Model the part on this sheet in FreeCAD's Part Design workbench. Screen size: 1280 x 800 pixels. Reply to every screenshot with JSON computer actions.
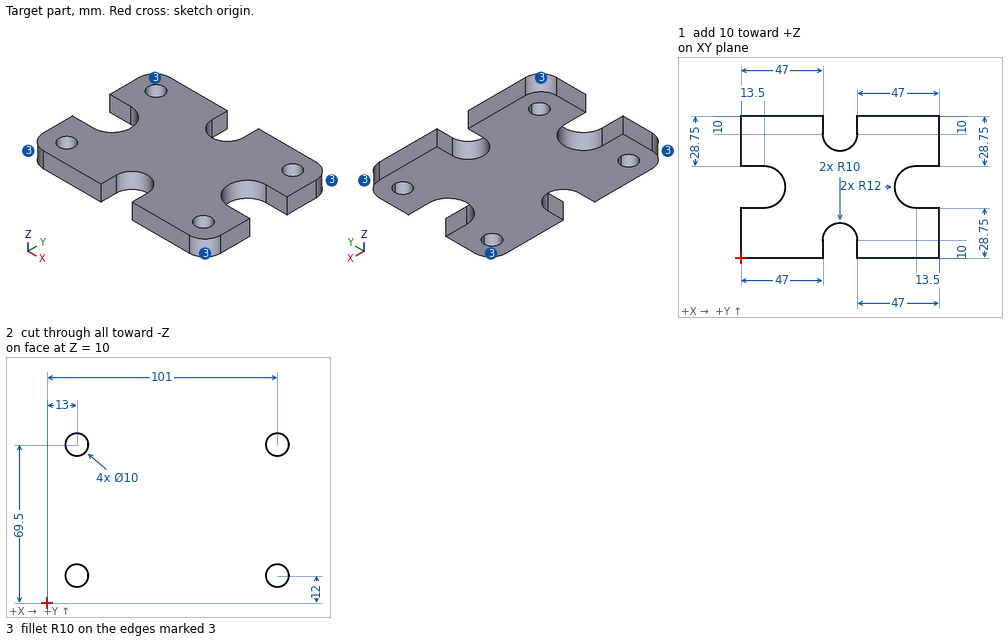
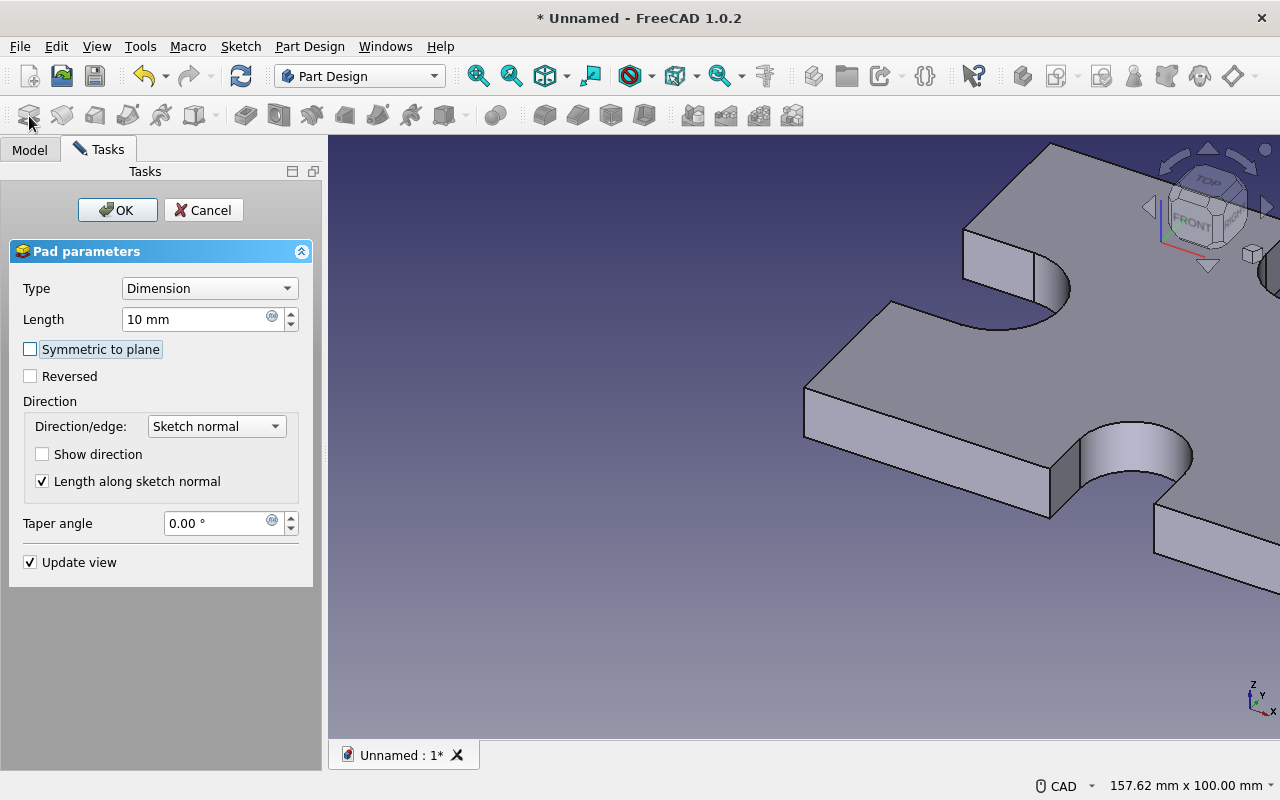
{"action": "left_click", "coordinate": [118, 210]}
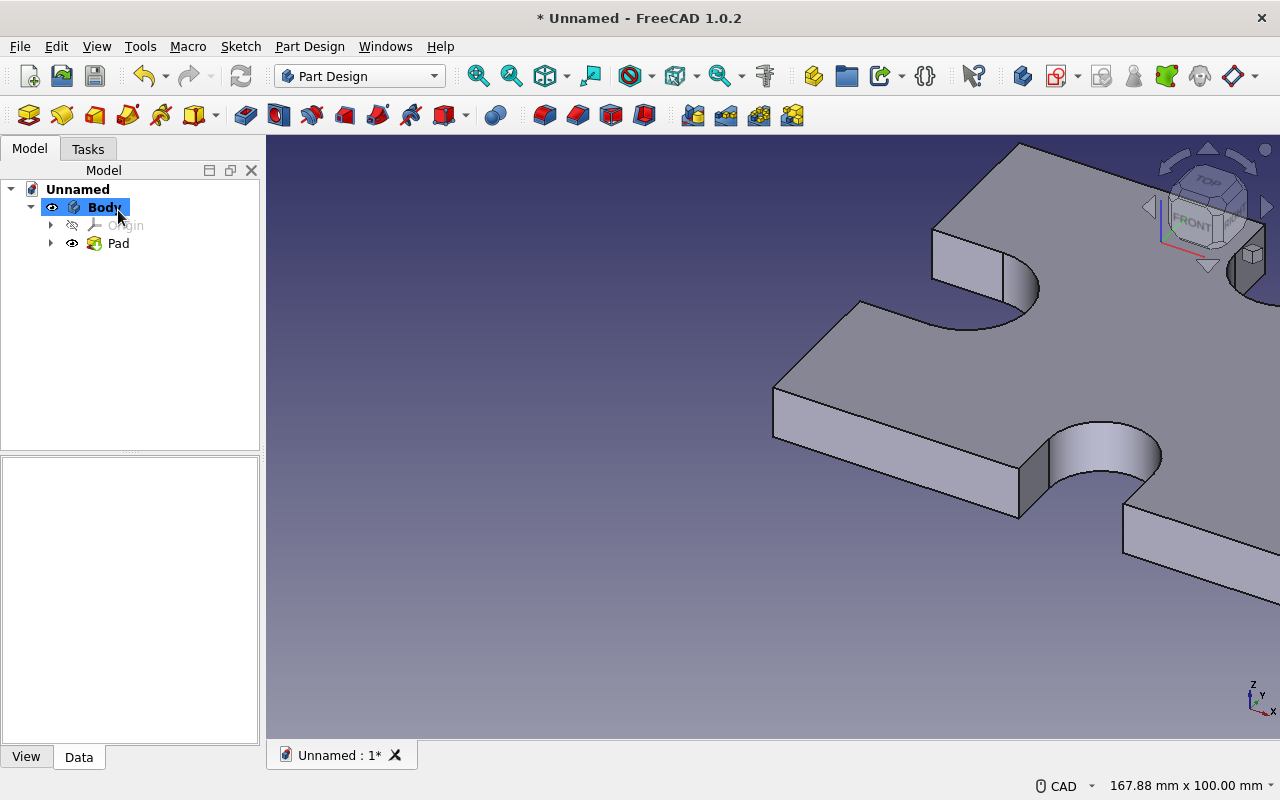
{"action": "left_click", "coordinate": [479, 76]}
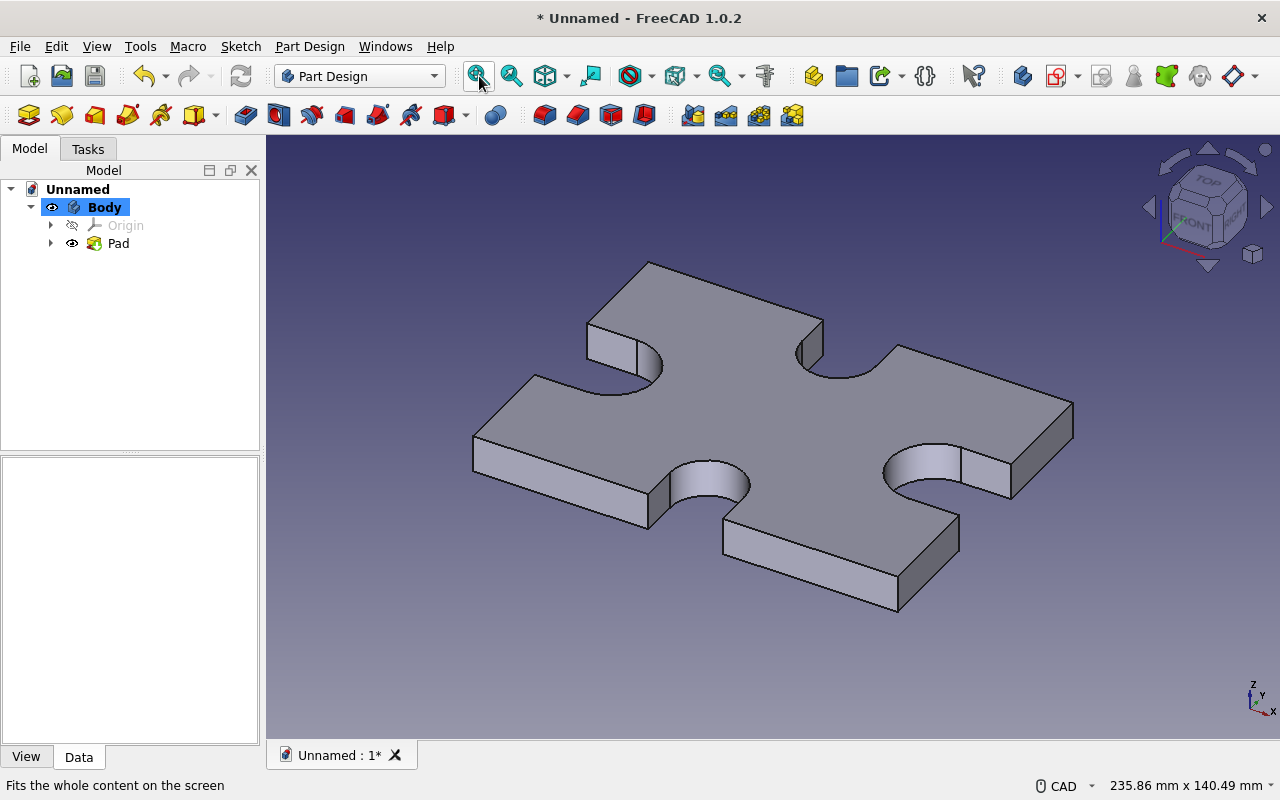
{"action": "left_click", "coordinate": [773, 418]}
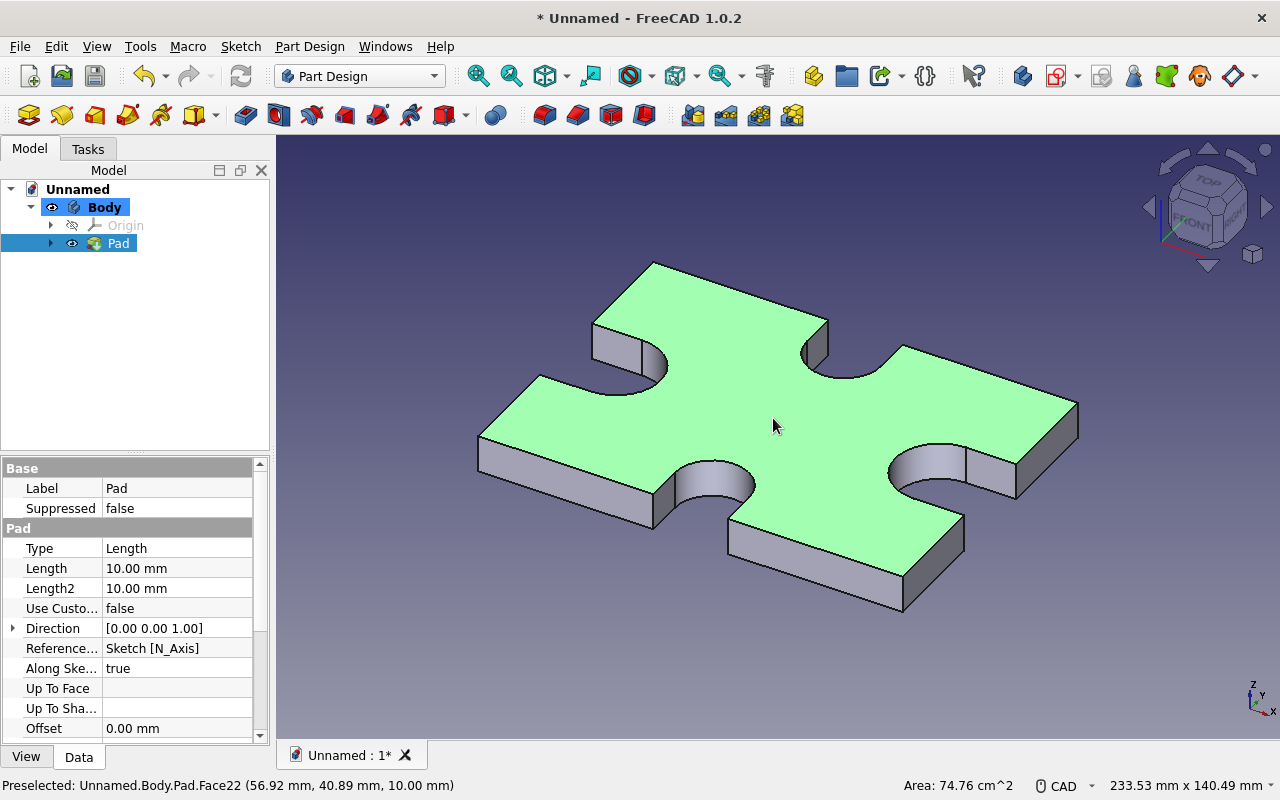
{"action": "left_click", "coordinate": [1056, 76]}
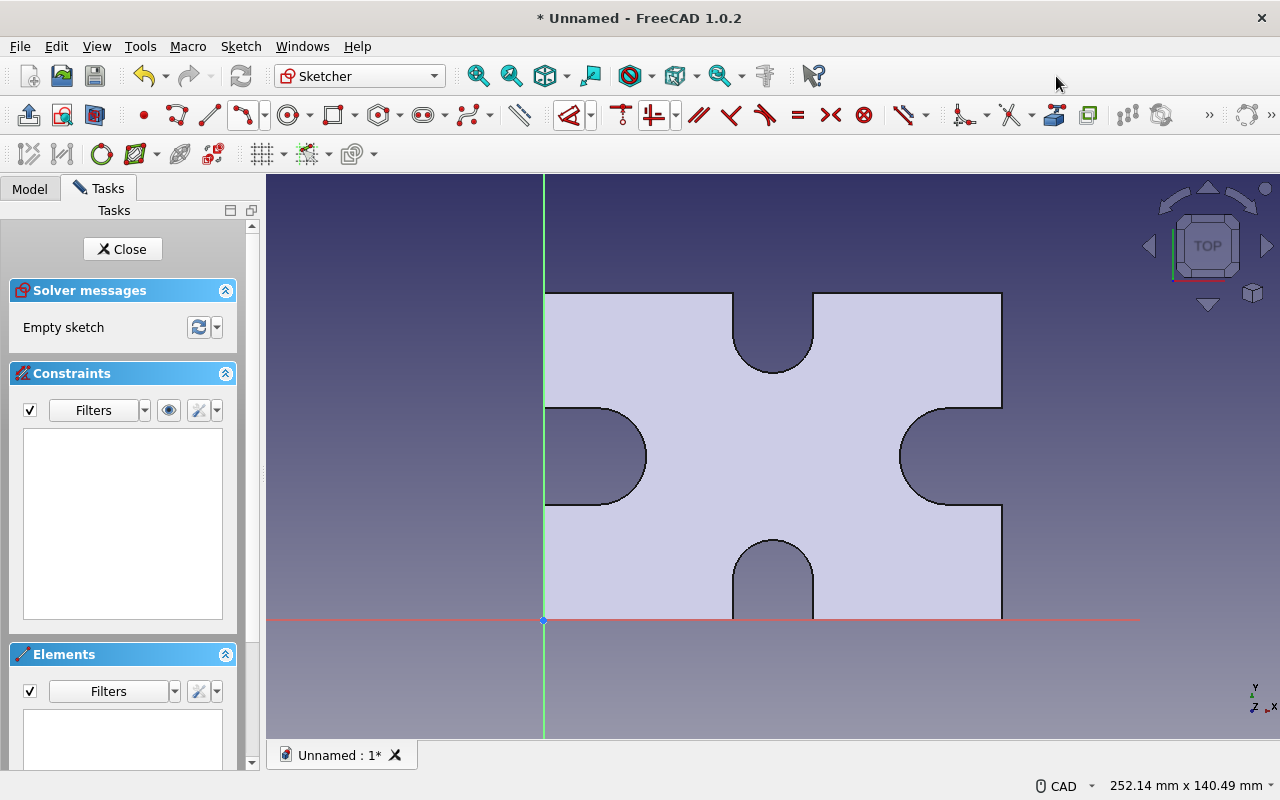
{"action": "left_click", "coordinate": [288, 116]}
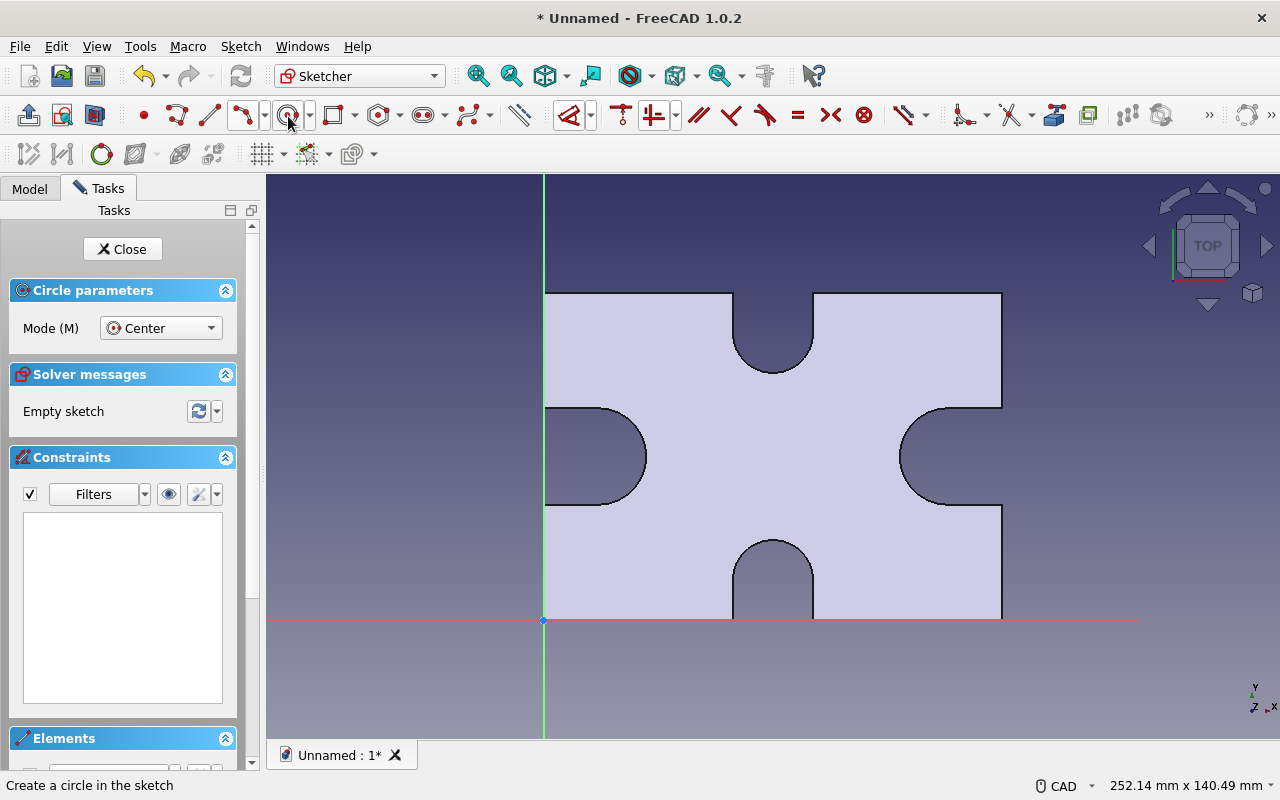
{"action": "left_click", "coordinate": [596, 341]}
{"action": "left_click", "coordinate": [610, 327]}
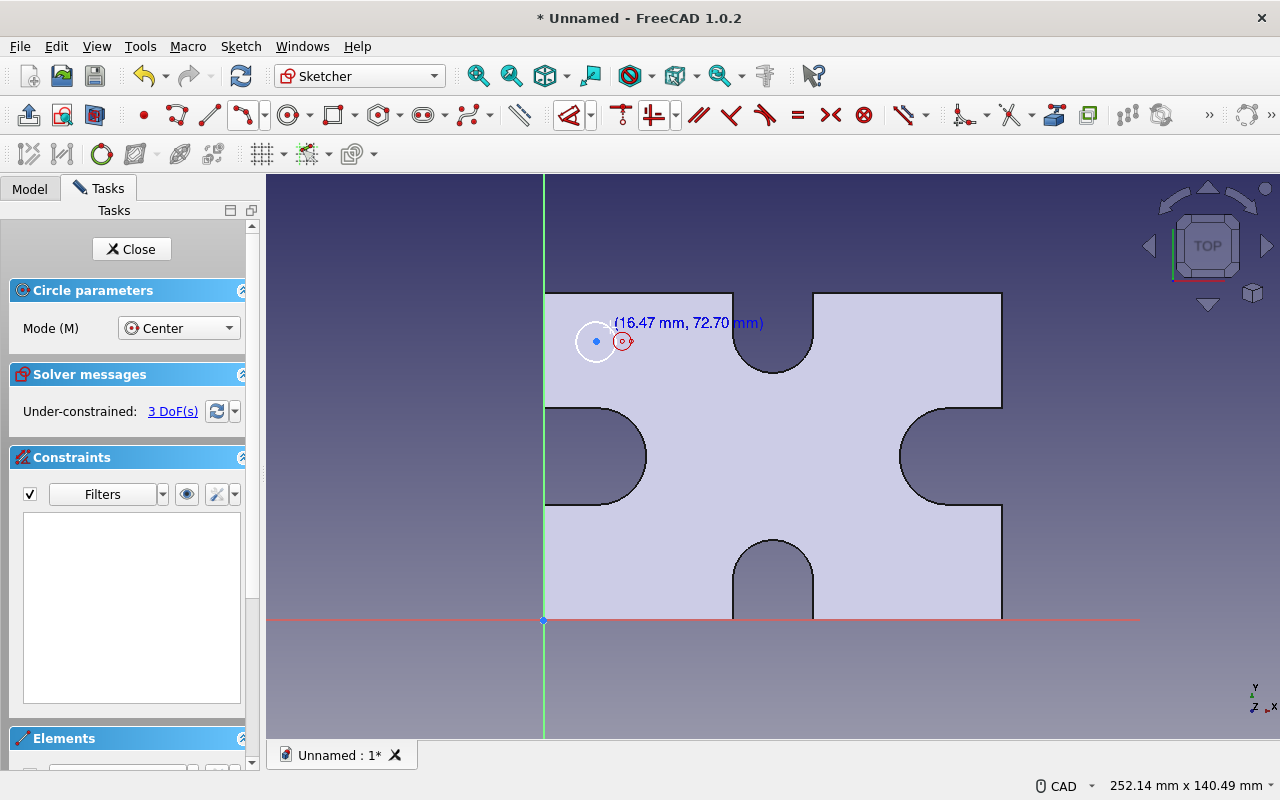
{"action": "left_click", "coordinate": [950, 341]}
{"action": "left_click", "coordinate": [964, 327]}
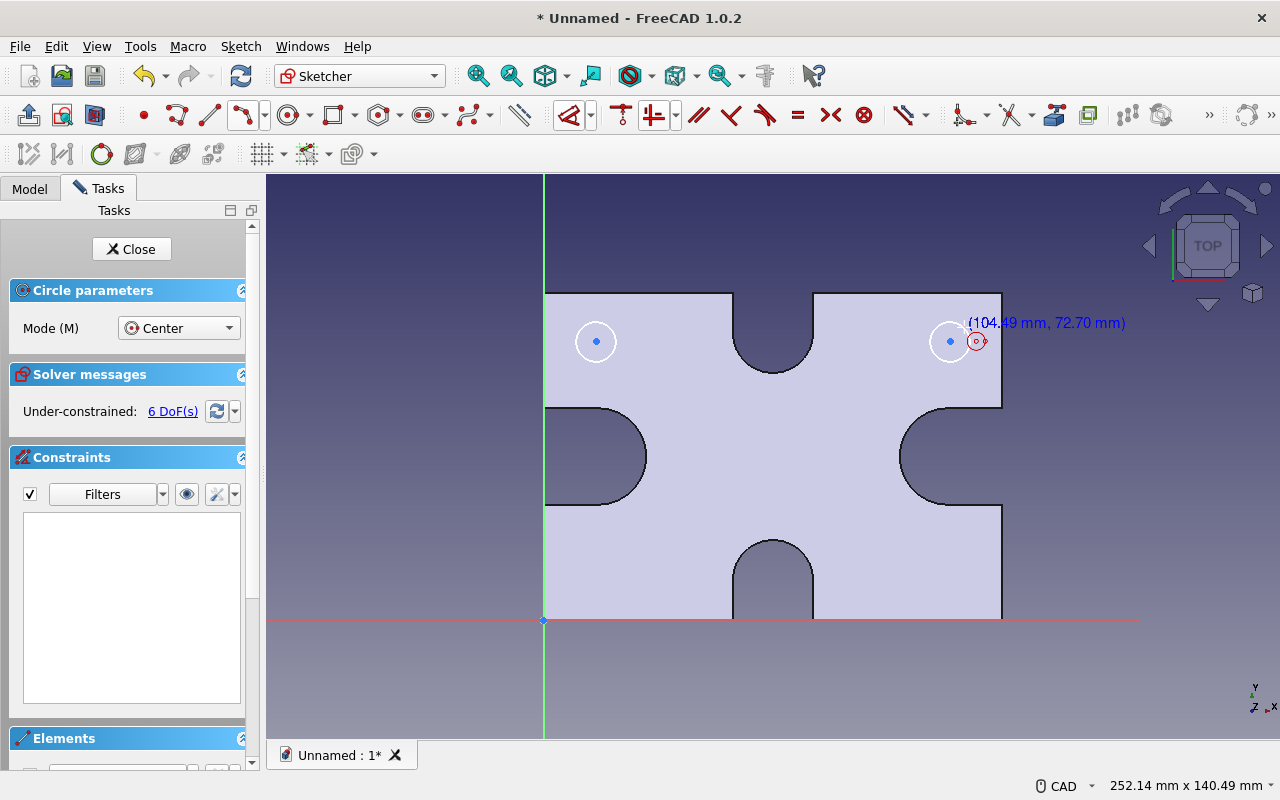
{"action": "left_click", "coordinate": [950, 572]}
{"action": "left_click", "coordinate": [964, 558]}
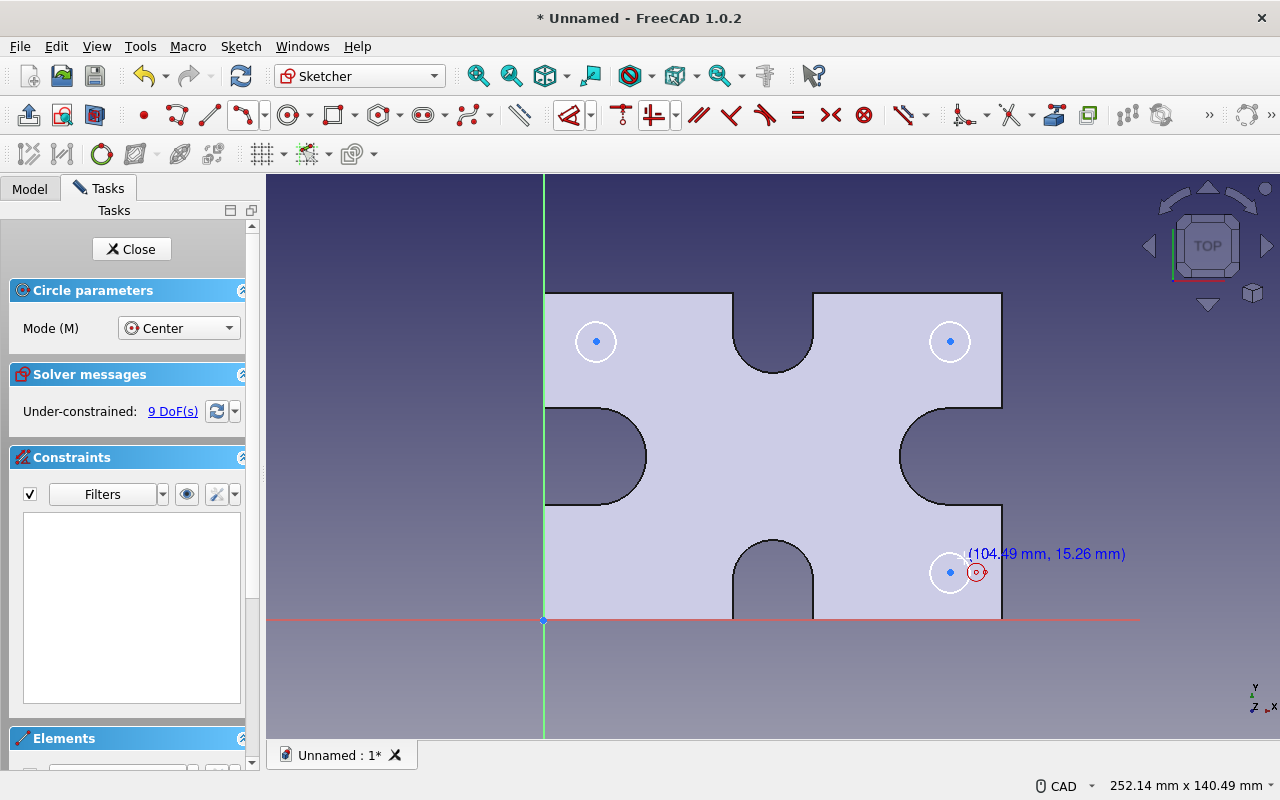
{"action": "left_click", "coordinate": [596, 572]}
{"action": "left_click", "coordinate": [610, 558]}
{"action": "key", "text": "Escape"}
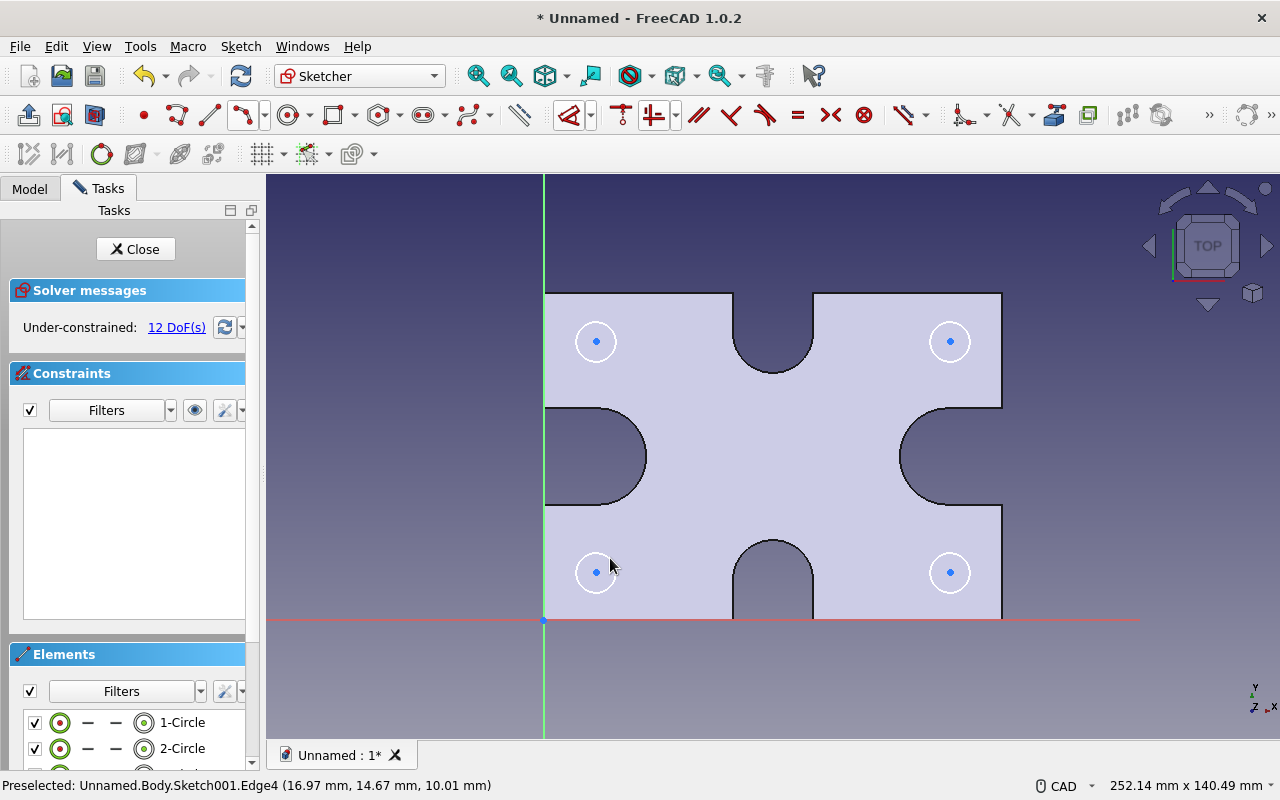
{"action": "left_click", "coordinate": [610, 328]}